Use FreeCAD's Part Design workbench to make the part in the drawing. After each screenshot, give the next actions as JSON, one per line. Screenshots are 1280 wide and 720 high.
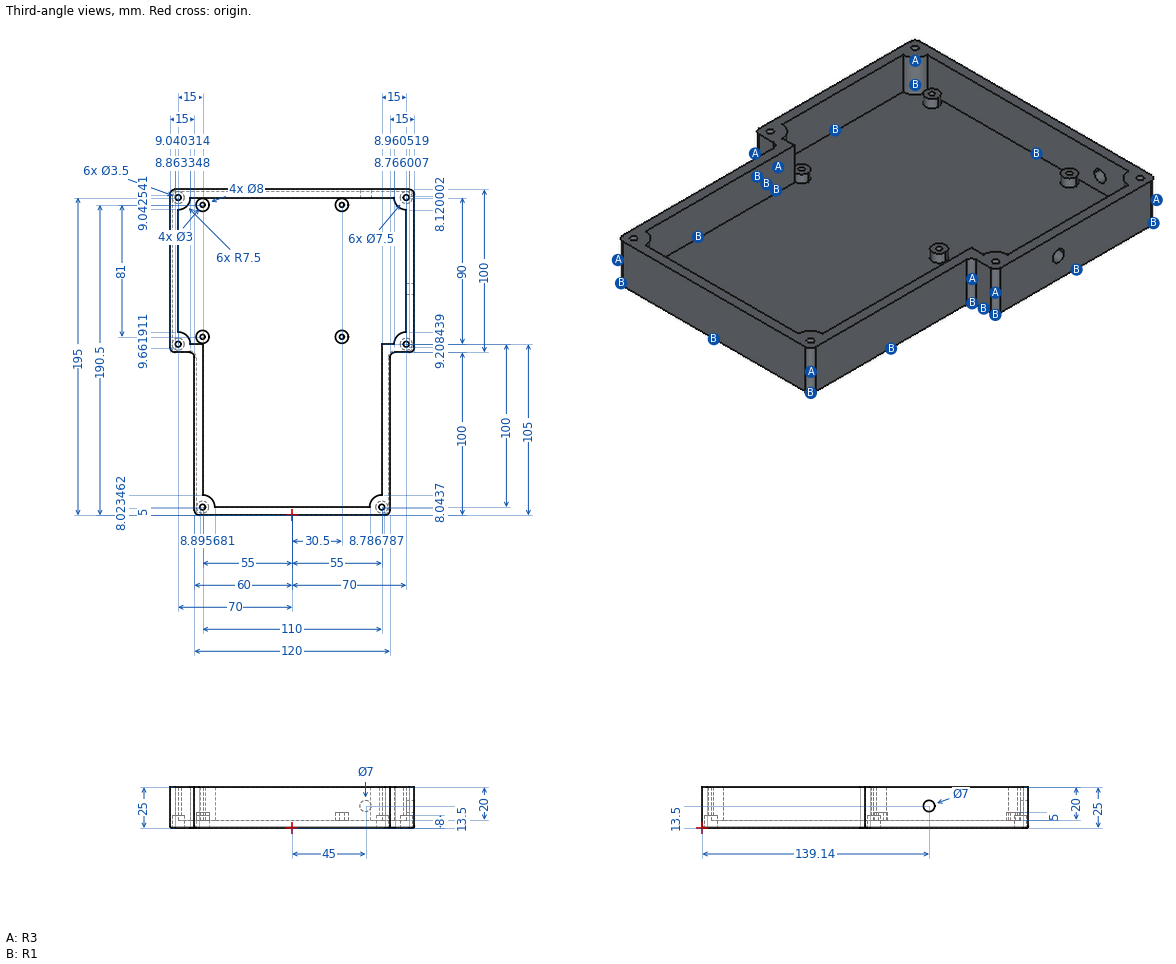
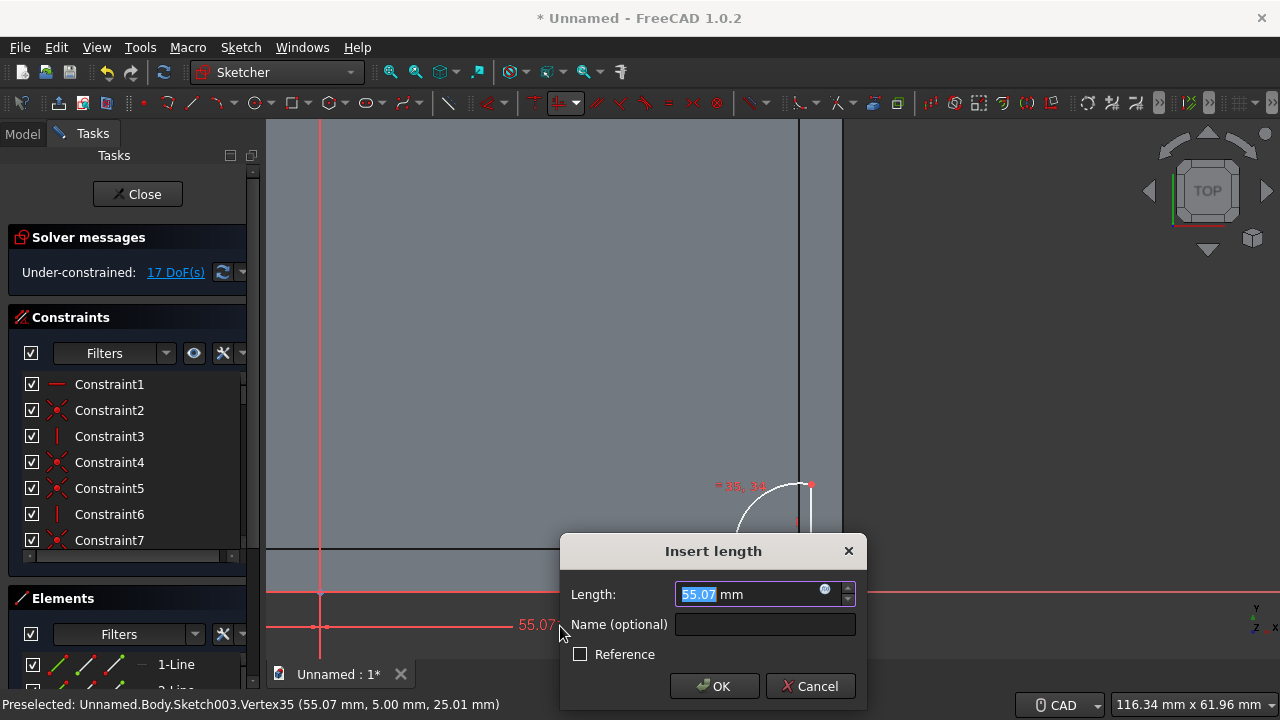
{"action": "type", "text": "55"}
{"action": "key", "text": "Return"}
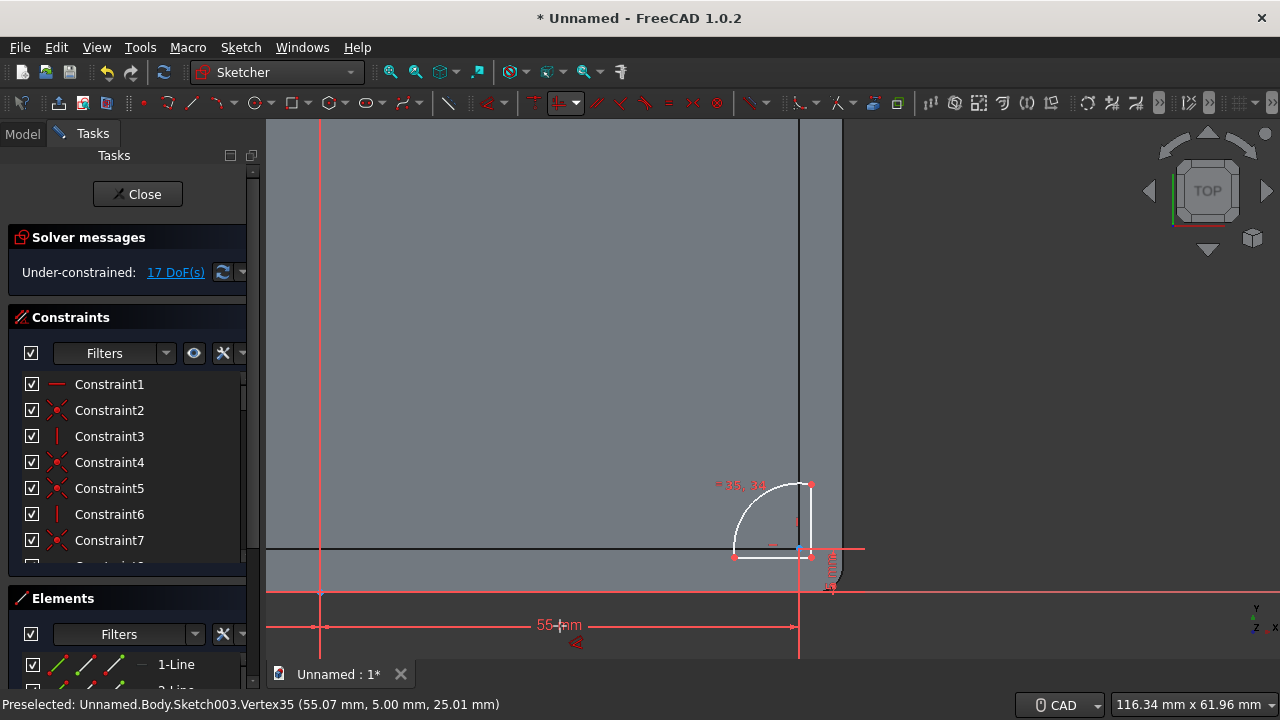
{"action": "scroll", "coordinate": [802, 554], "scroll_direction": "down", "scroll_amount": 8}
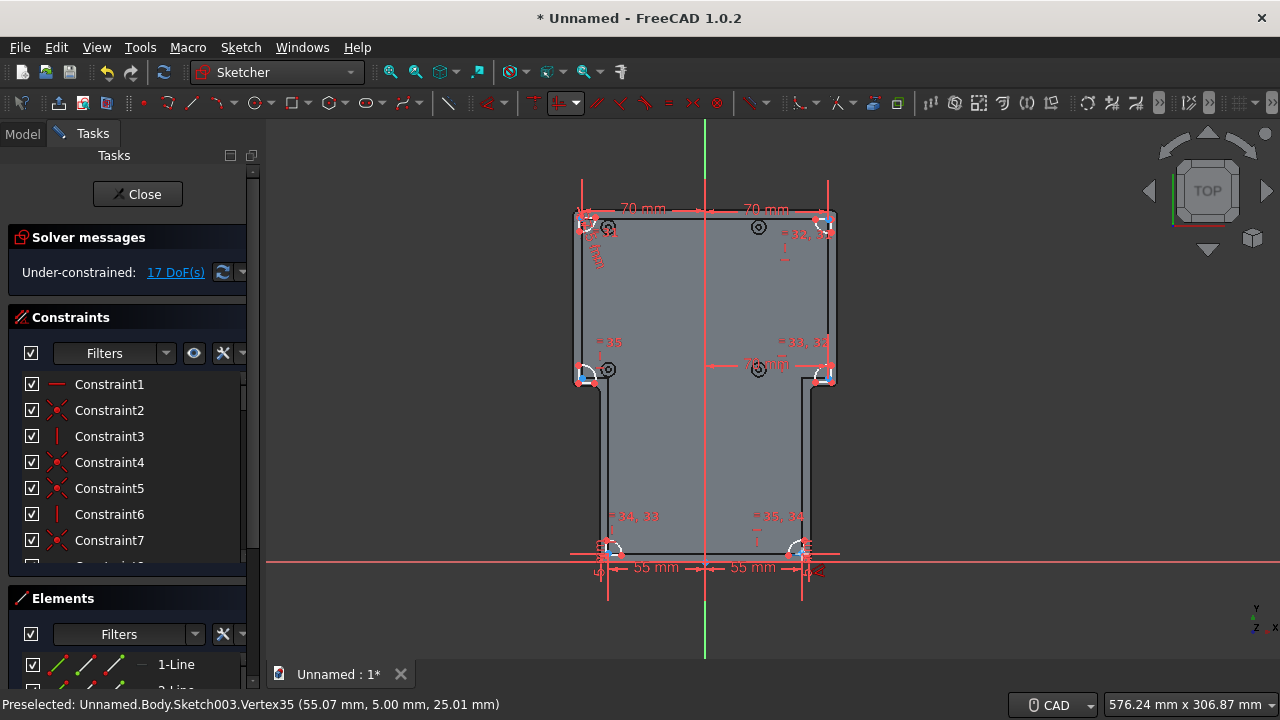
{"action": "scroll", "coordinate": [582, 379], "scroll_direction": "up", "scroll_amount": 4}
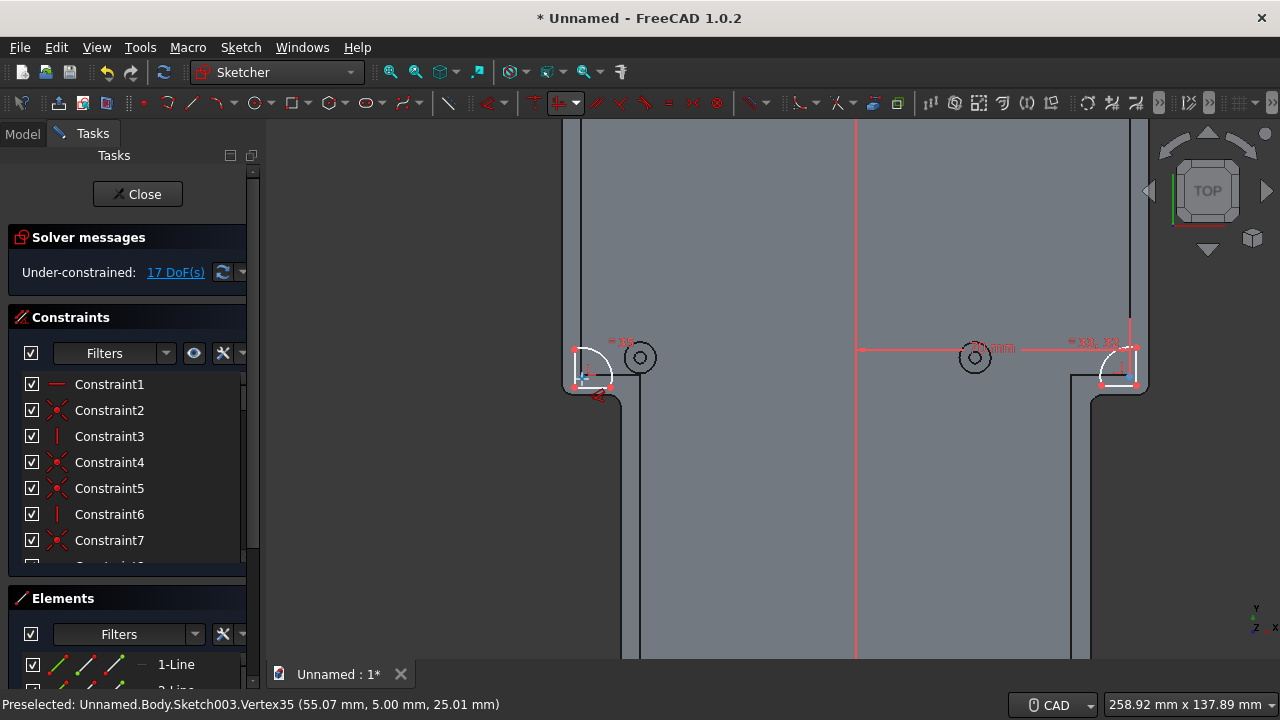
{"action": "left_click", "coordinate": [583, 377]}
{"action": "left_click", "coordinate": [719, 343]}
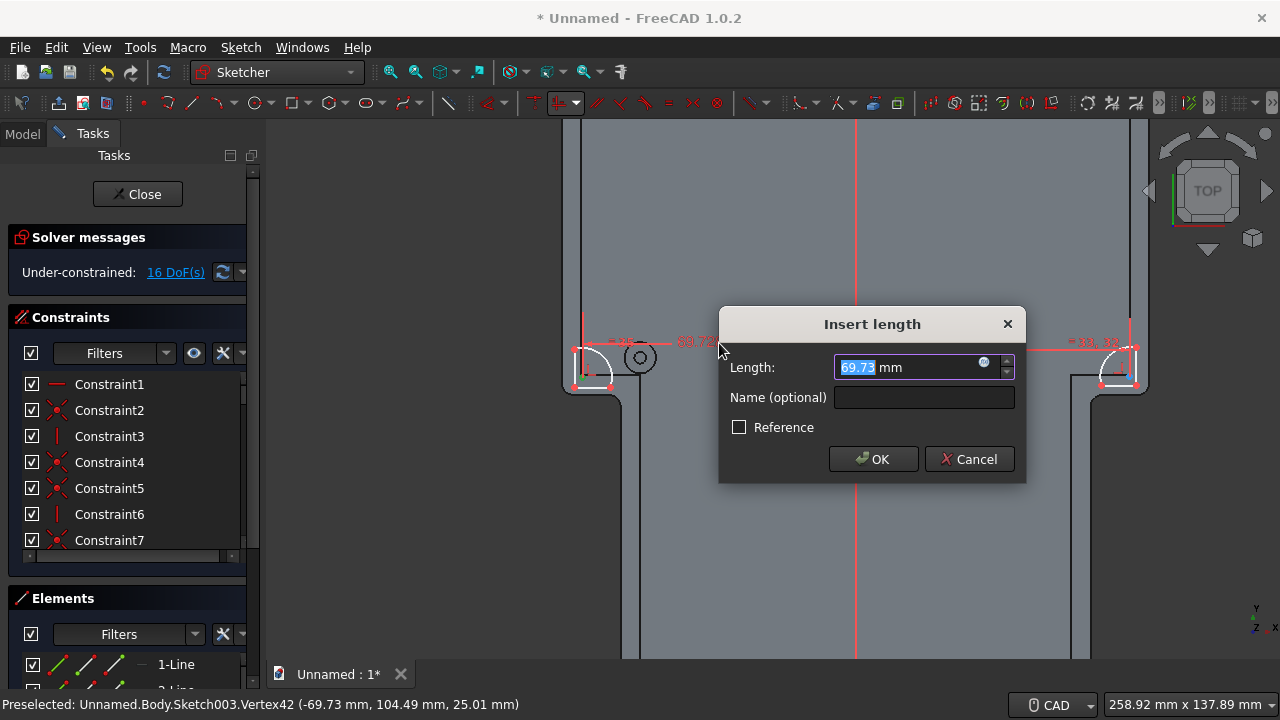
{"action": "type", "text": "70"}
{"action": "key", "text": "Return"}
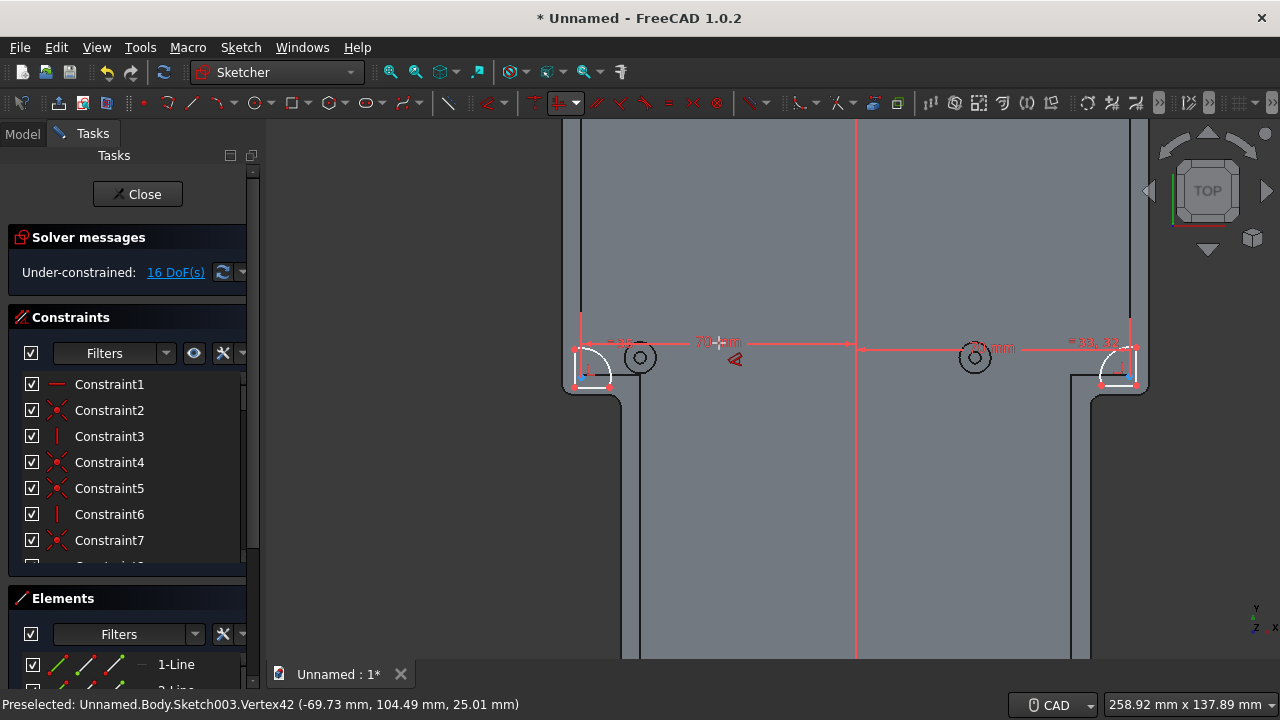
{"action": "scroll", "coordinate": [582, 379], "scroll_direction": "down", "scroll_amount": 4}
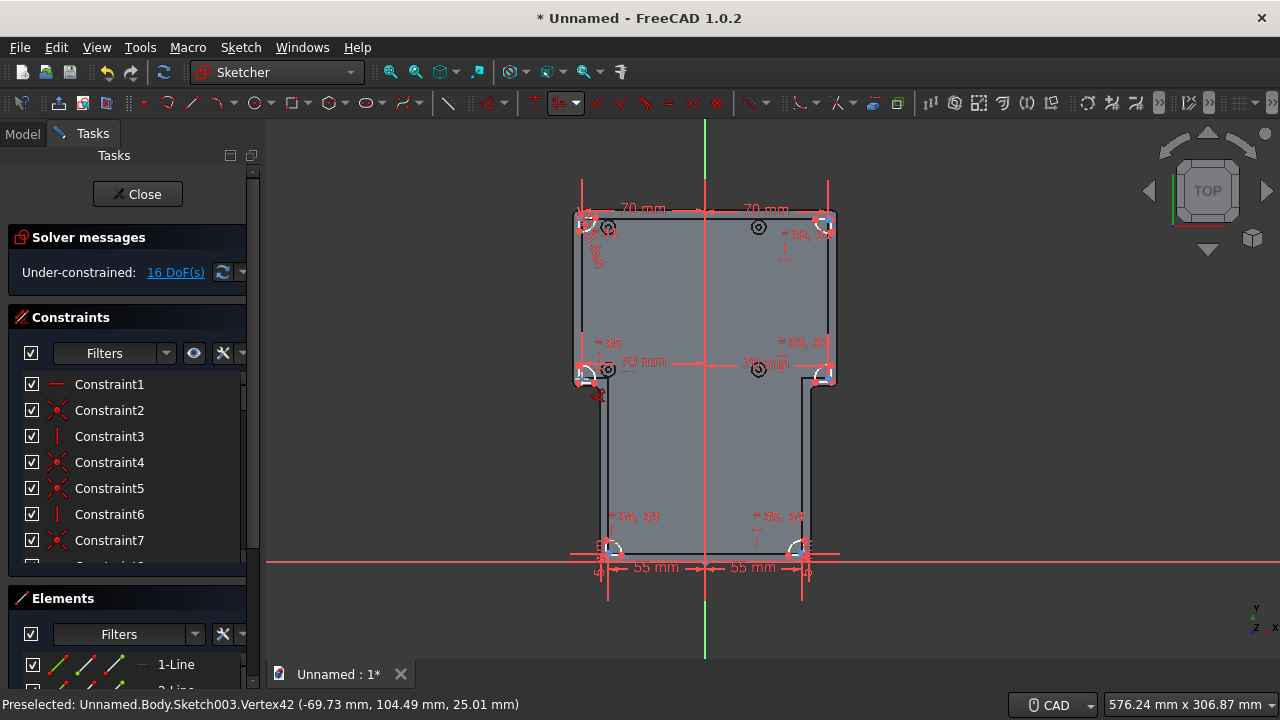
{"action": "scroll", "coordinate": [582, 219], "scroll_direction": "up", "scroll_amount": 8}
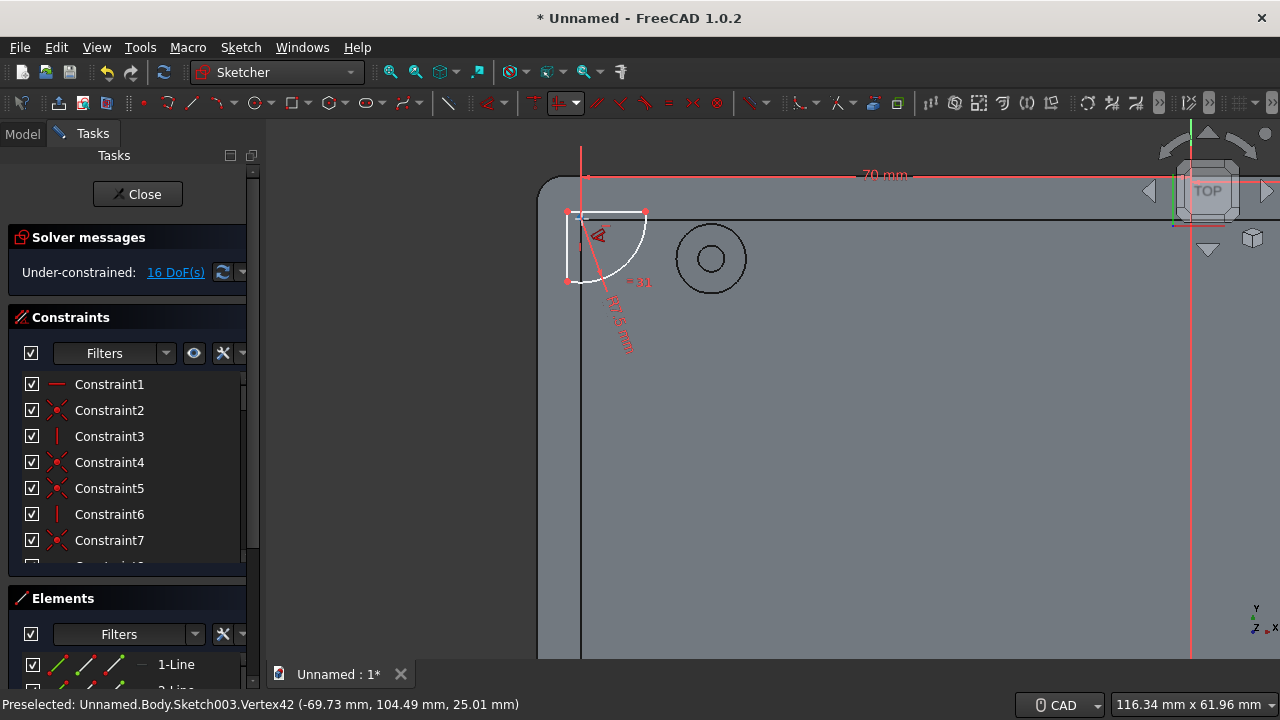
{"action": "left_click", "coordinate": [581, 217]}
{"action": "left_click", "coordinate": [547, 424]}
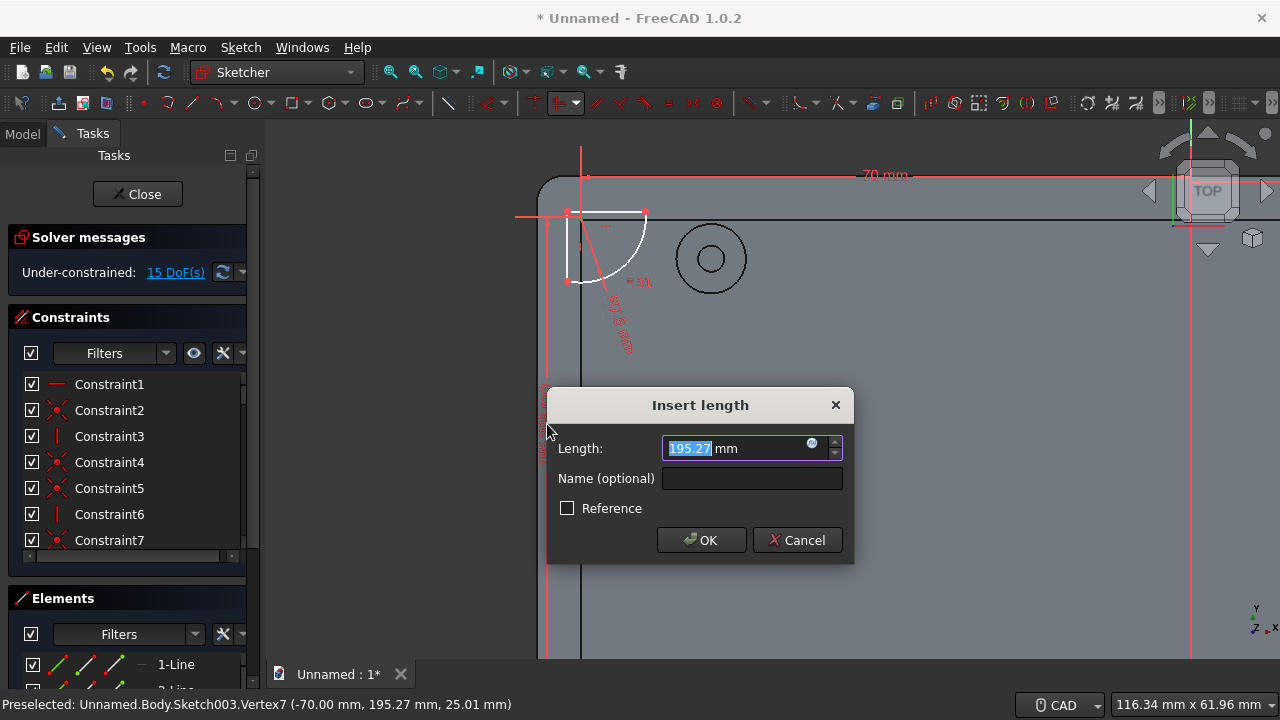
{"action": "type", "text": "195"}
{"action": "key", "text": "Return"}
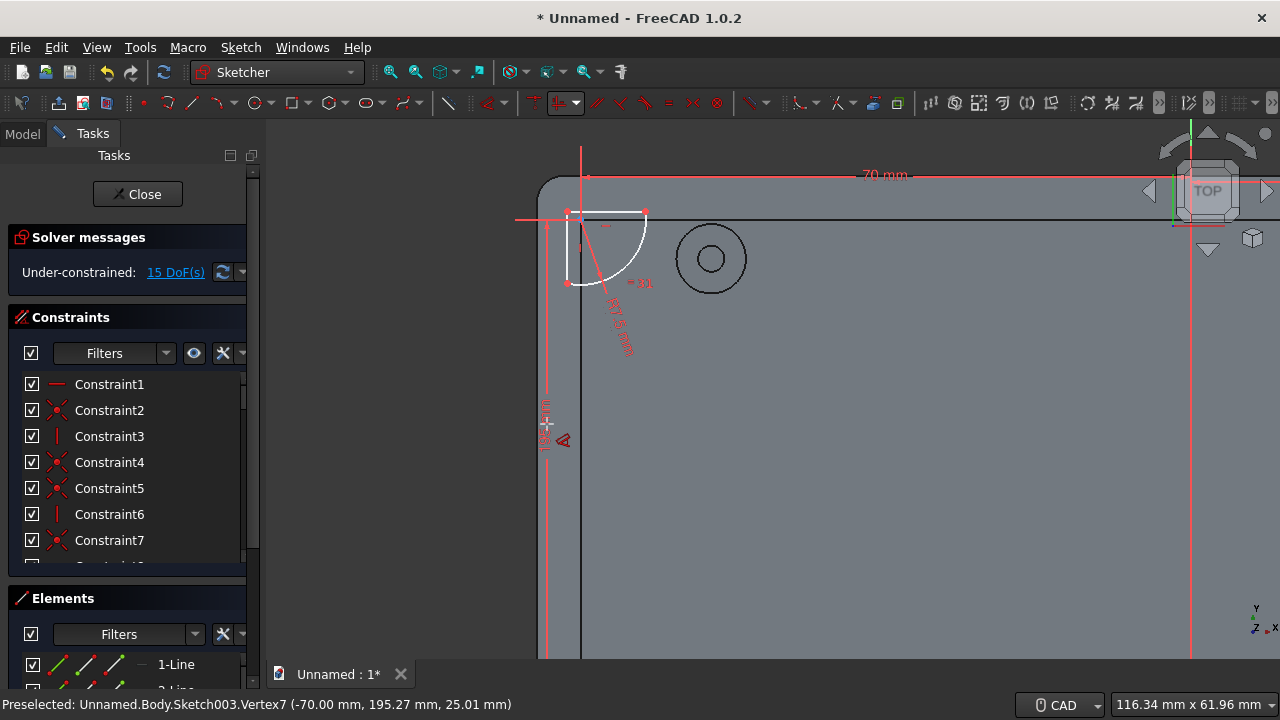
{"action": "scroll", "coordinate": [582, 219], "scroll_direction": "down", "scroll_amount": 8}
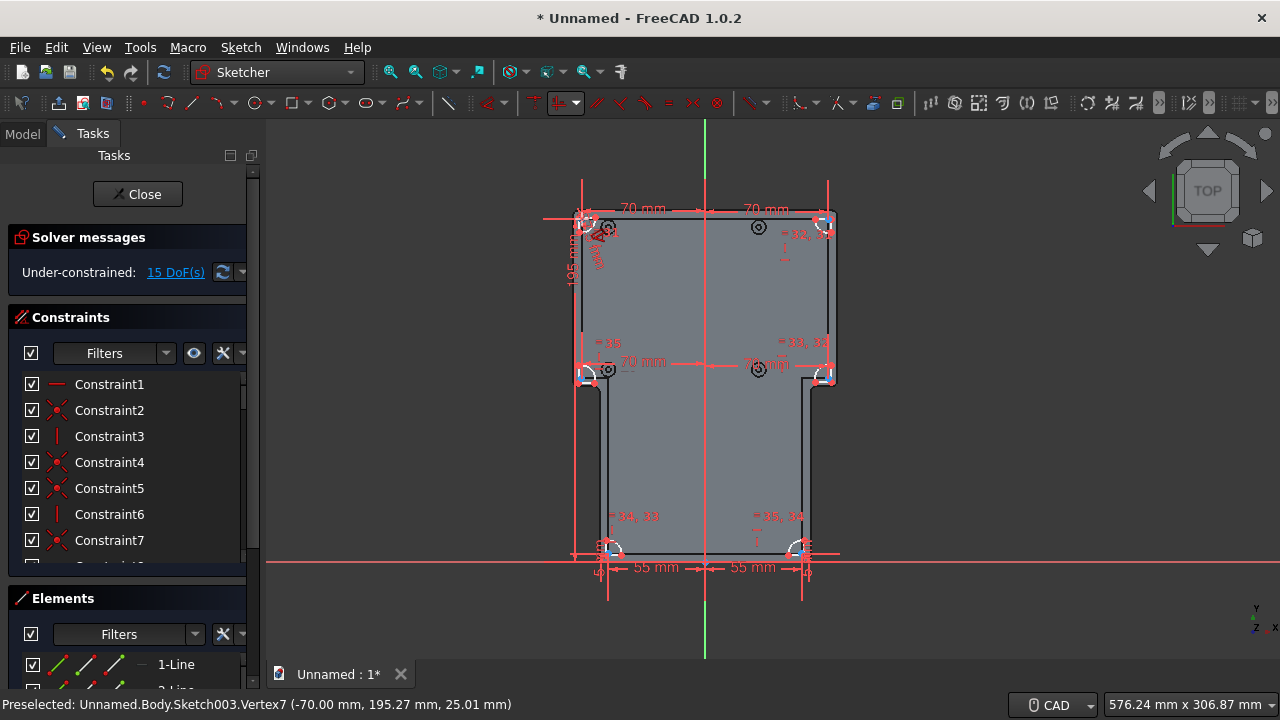
{"action": "scroll", "coordinate": [828, 220], "scroll_direction": "up", "scroll_amount": 8}